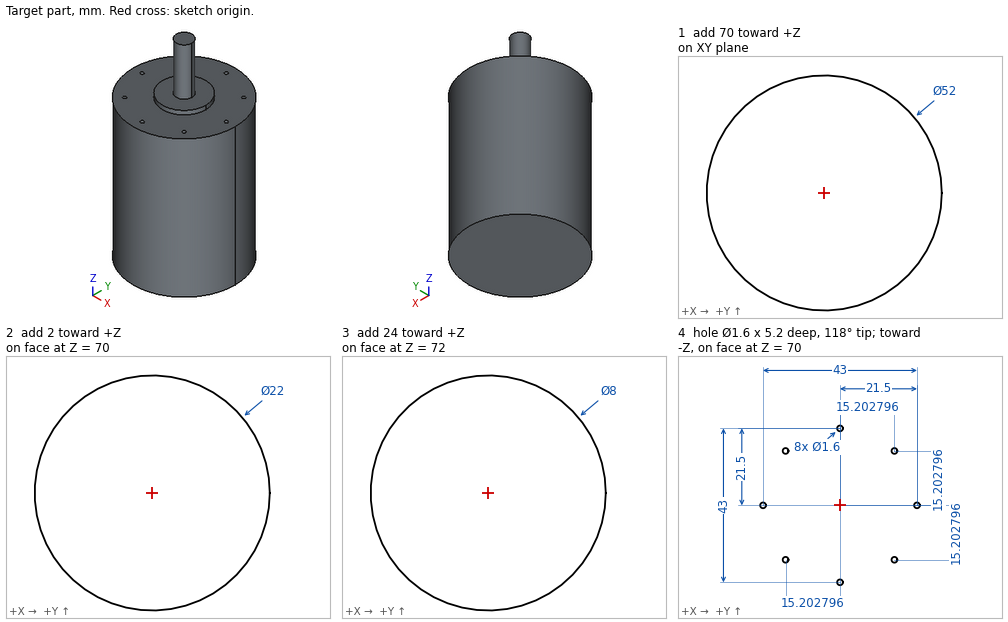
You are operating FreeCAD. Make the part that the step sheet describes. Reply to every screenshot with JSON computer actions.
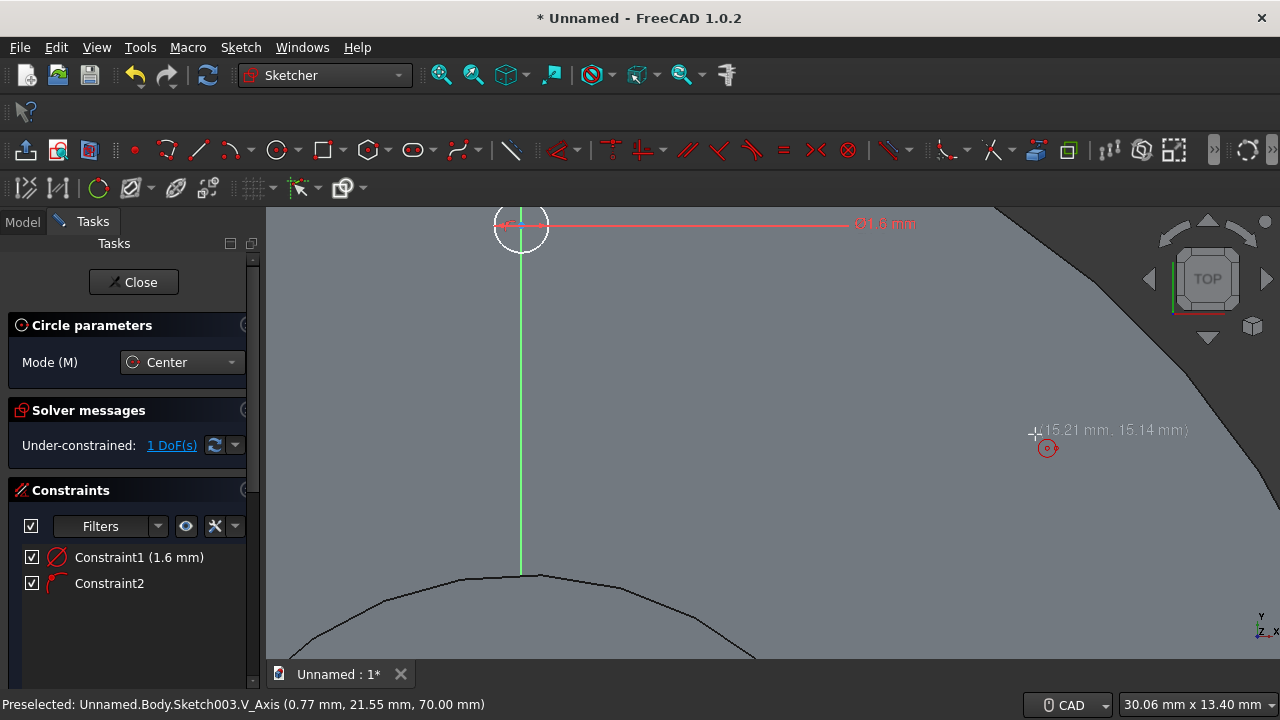
{"action": "scroll", "coordinate": [751, 303], "scroll_direction": "down", "scroll_amount": 8}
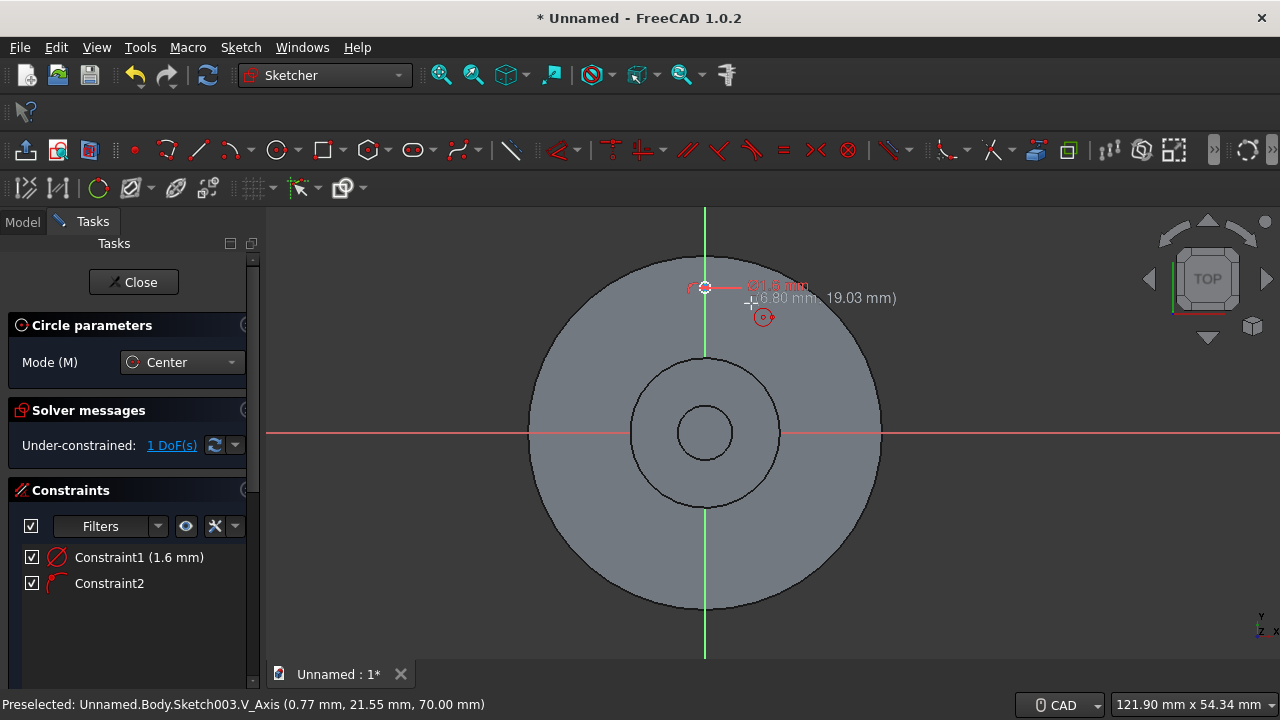
{"action": "left_click", "coordinate": [809, 329]}
{"action": "mouse_move", "coordinate": [812, 326]}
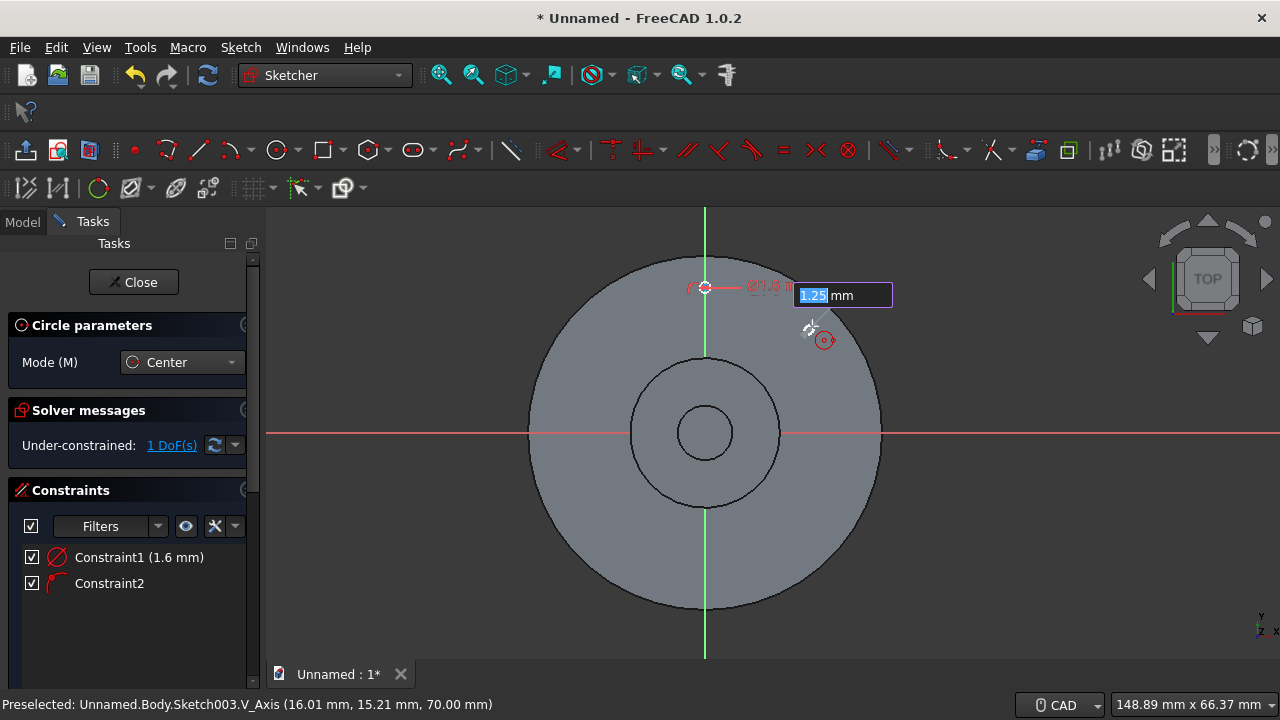
{"action": "type", "text": "1.6"}
{"action": "key", "text": "Return"}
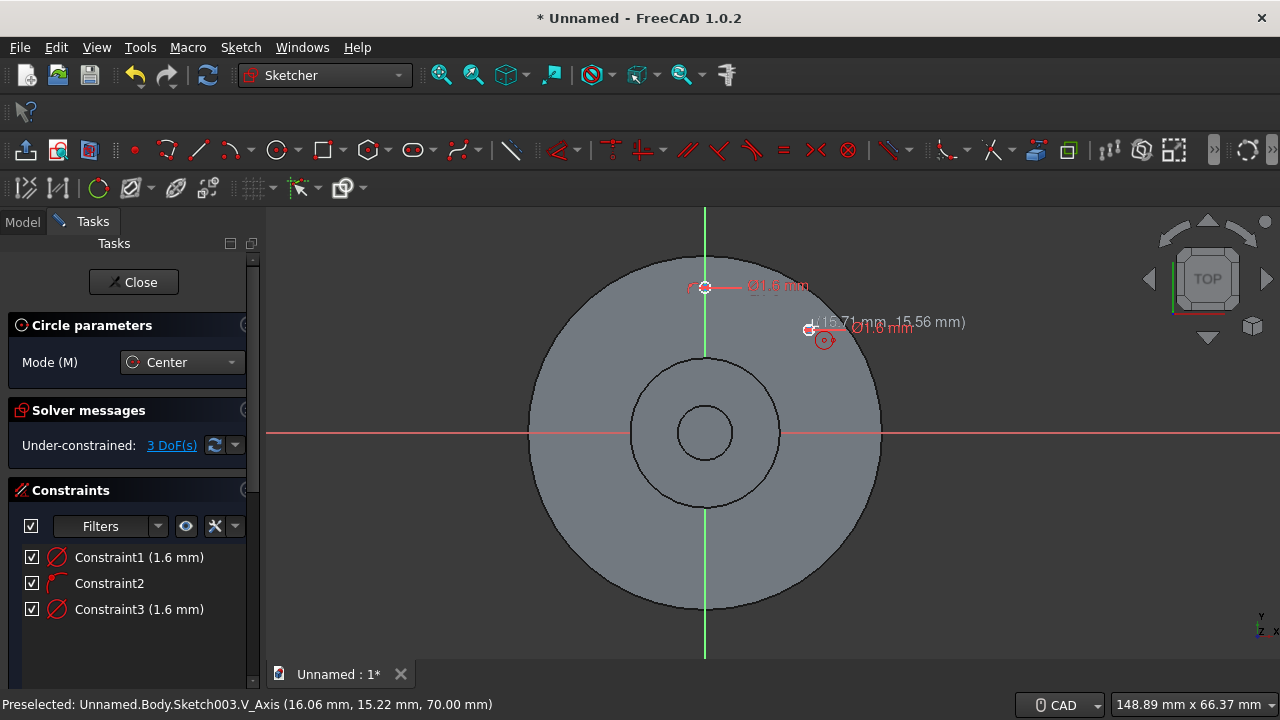
{"action": "scroll", "coordinate": [851, 433], "scroll_direction": "up", "scroll_amount": 8}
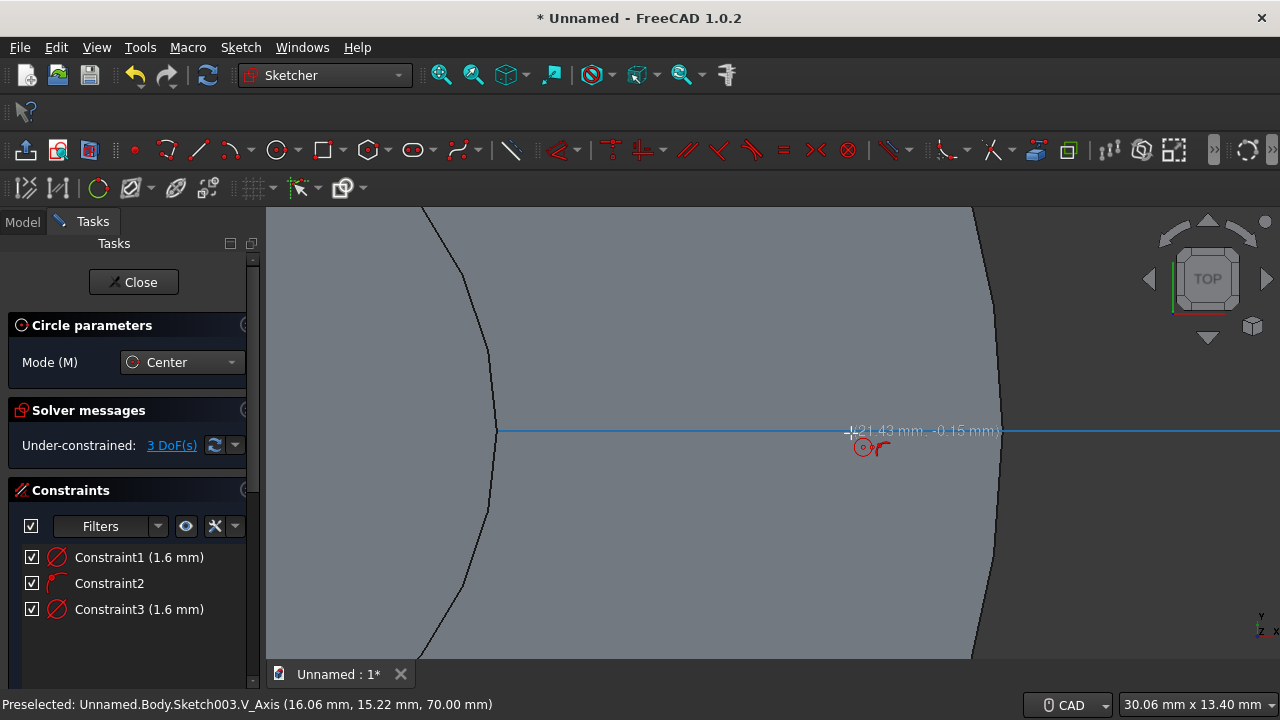
{"action": "scroll", "coordinate": [851, 434], "scroll_direction": "down", "scroll_amount": 8}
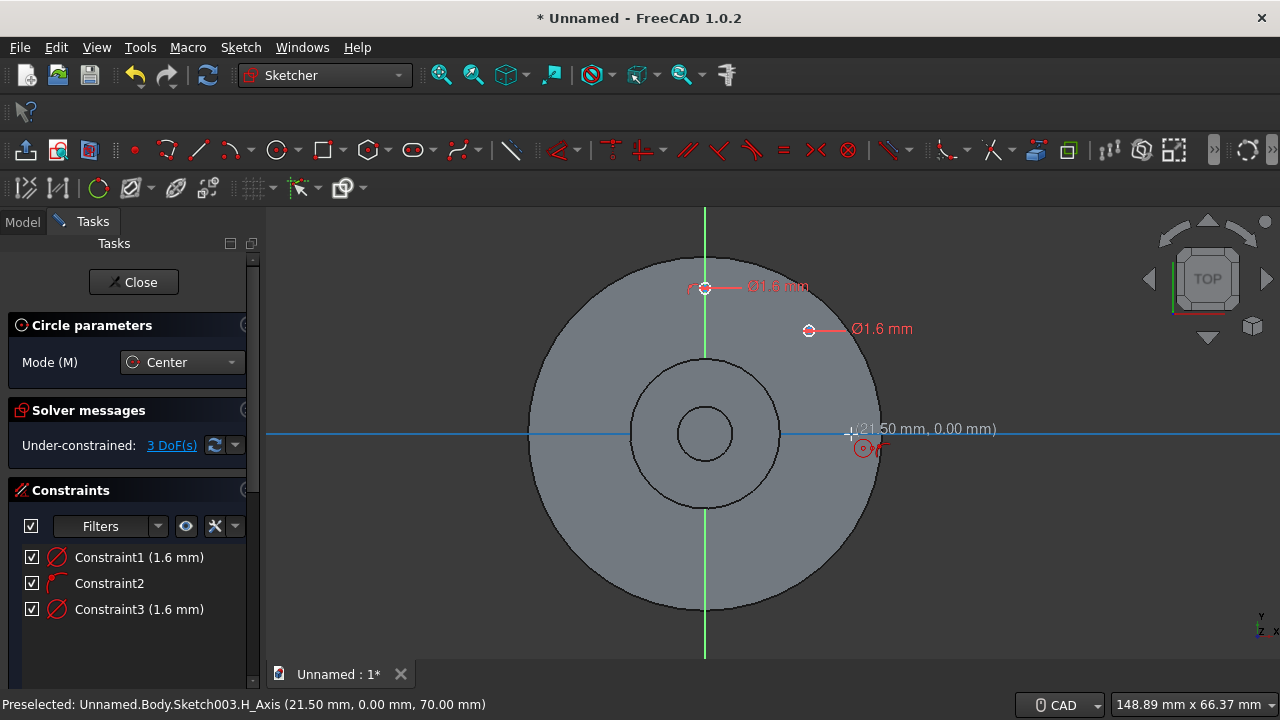
{"action": "left_click", "coordinate": [851, 434]}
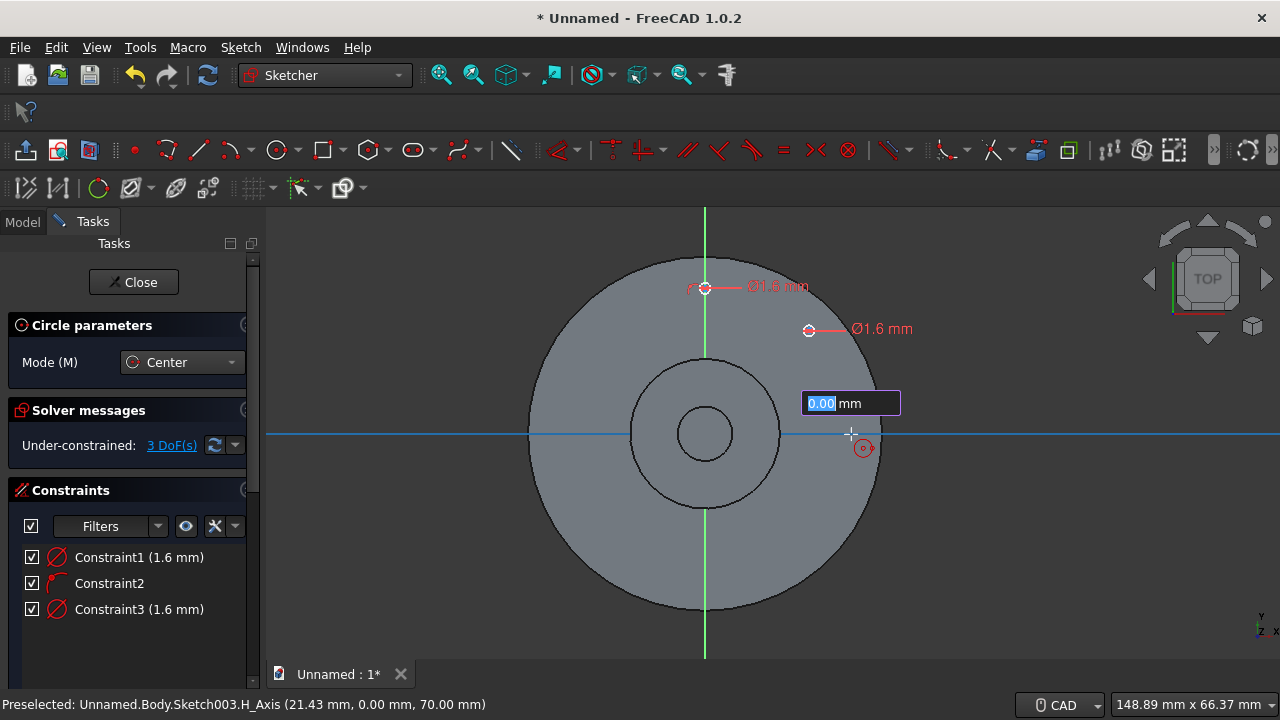
{"action": "scroll", "coordinate": [850, 439], "scroll_direction": "up", "scroll_amount": 6}
{"action": "mouse_move", "coordinate": [847, 437]}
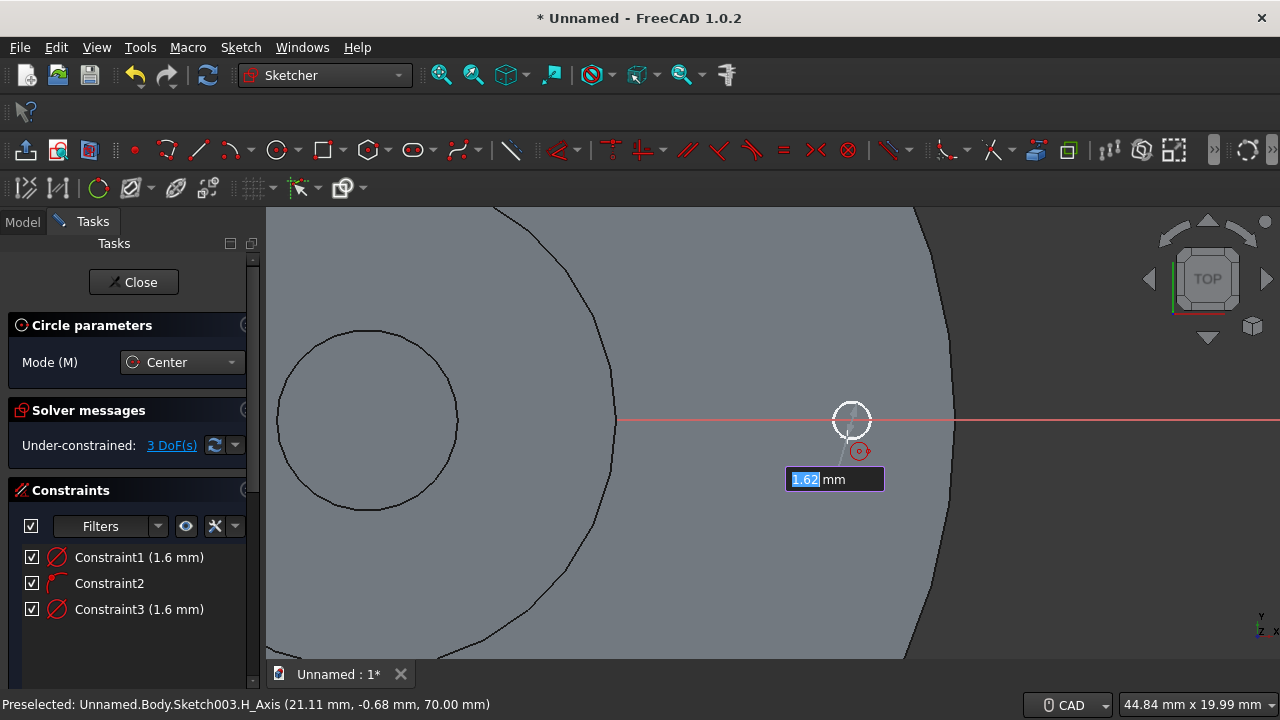
{"action": "type", "text": "1.6"}
{"action": "key", "text": "Return"}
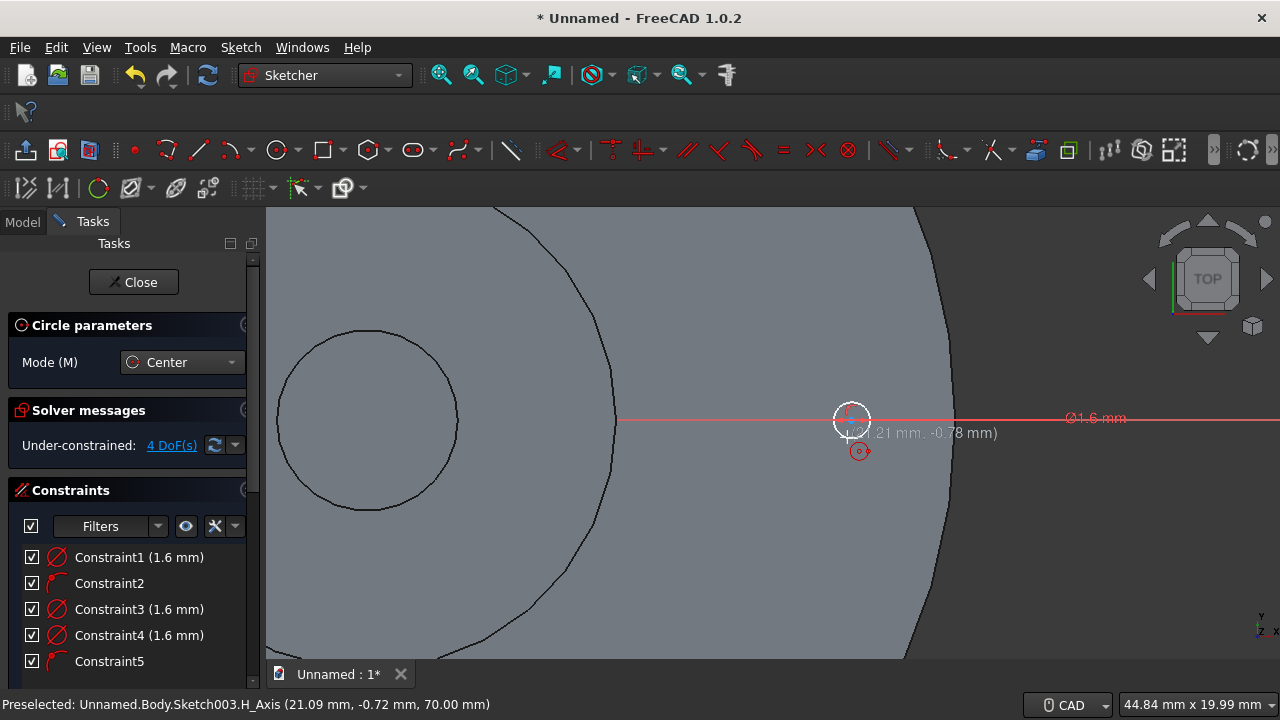
{"action": "scroll", "coordinate": [850, 438], "scroll_direction": "down", "scroll_amount": 6}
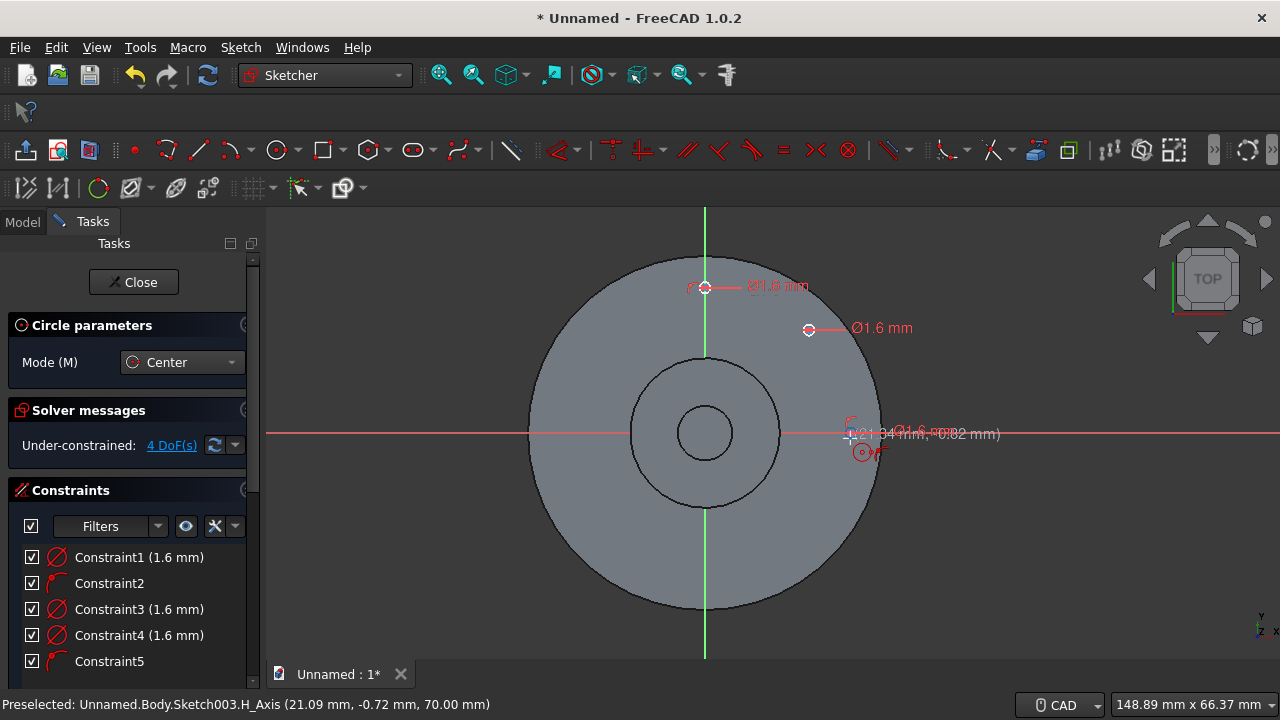
{"action": "scroll", "coordinate": [809, 537], "scroll_direction": "up", "scroll_amount": 8}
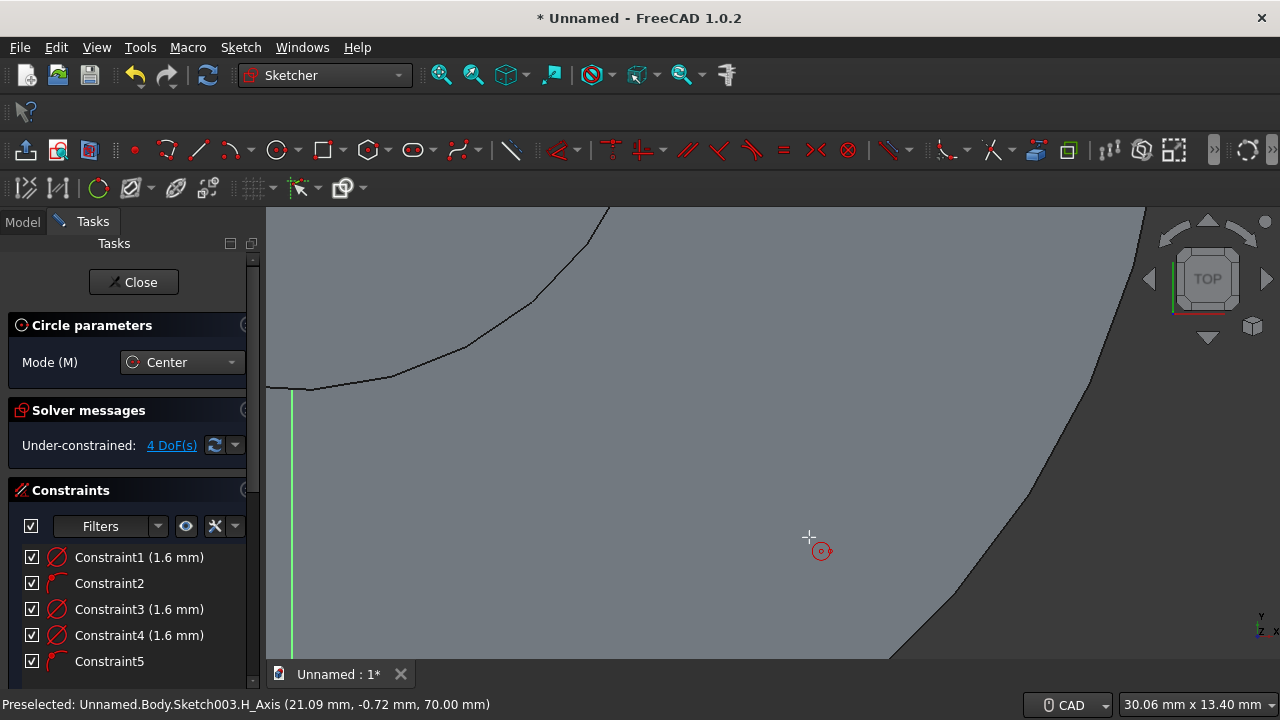
{"action": "scroll", "coordinate": [809, 538], "scroll_direction": "down", "scroll_amount": 8}